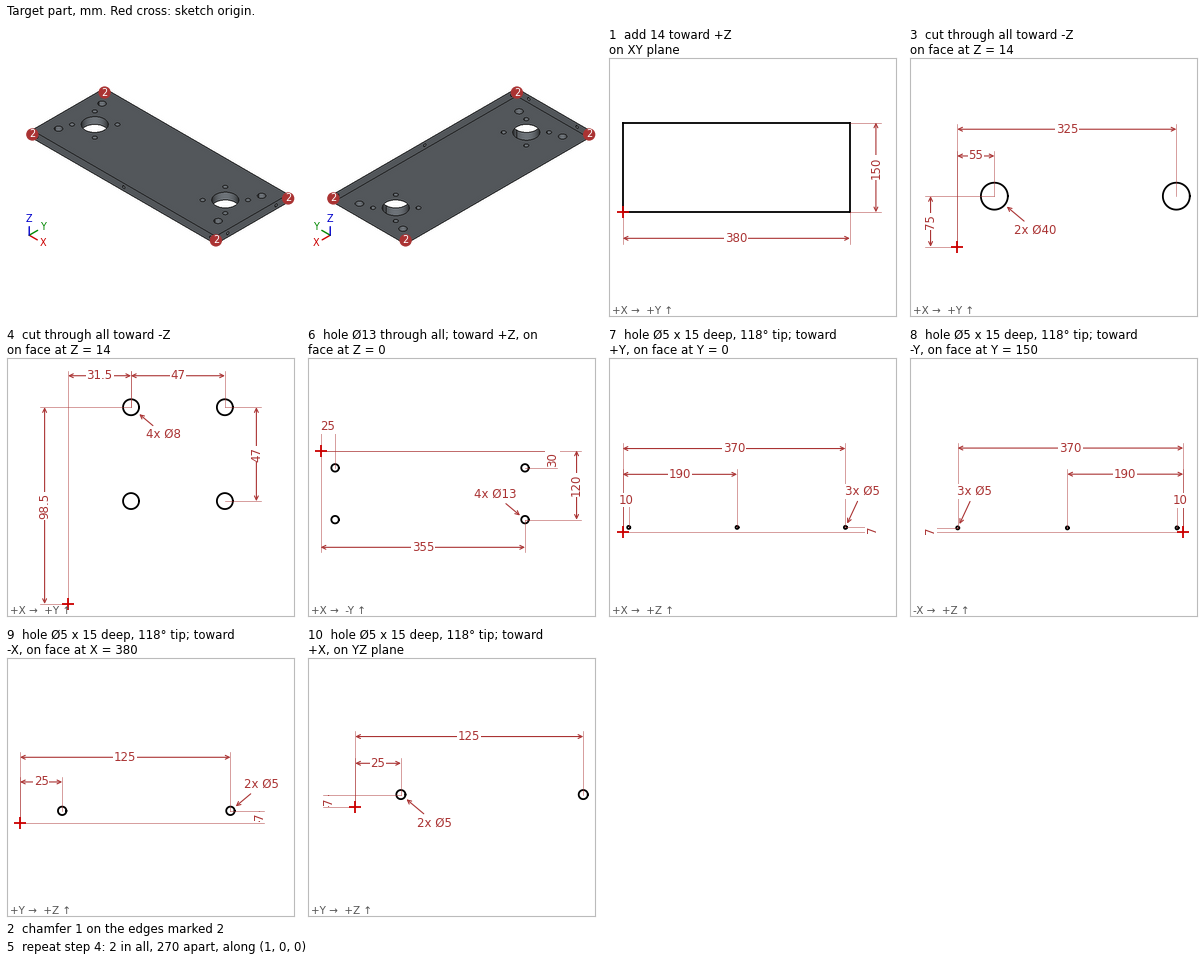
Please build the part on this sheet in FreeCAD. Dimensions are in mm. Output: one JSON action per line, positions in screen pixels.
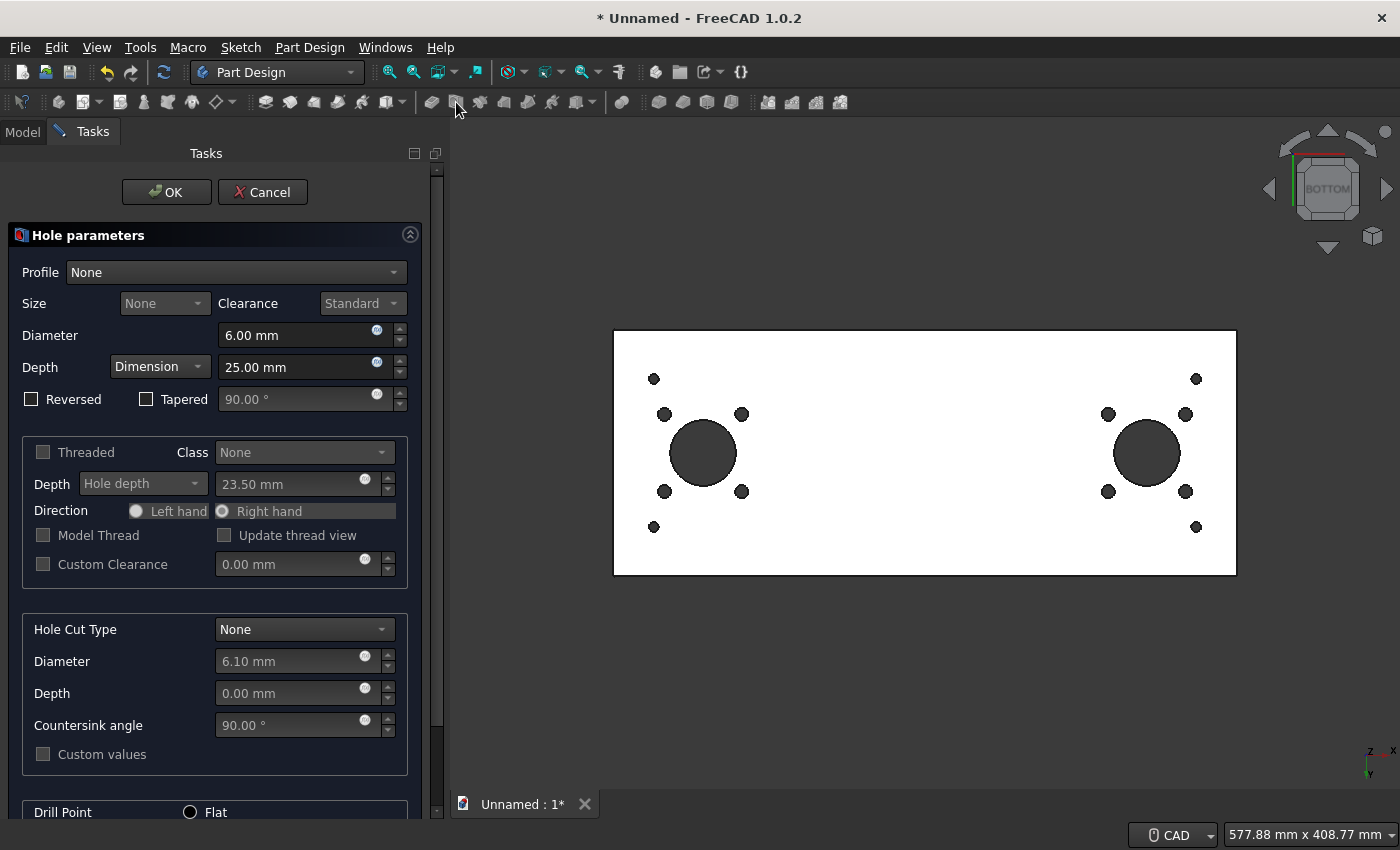
{"action": "triple_click", "coordinate": [305, 335]}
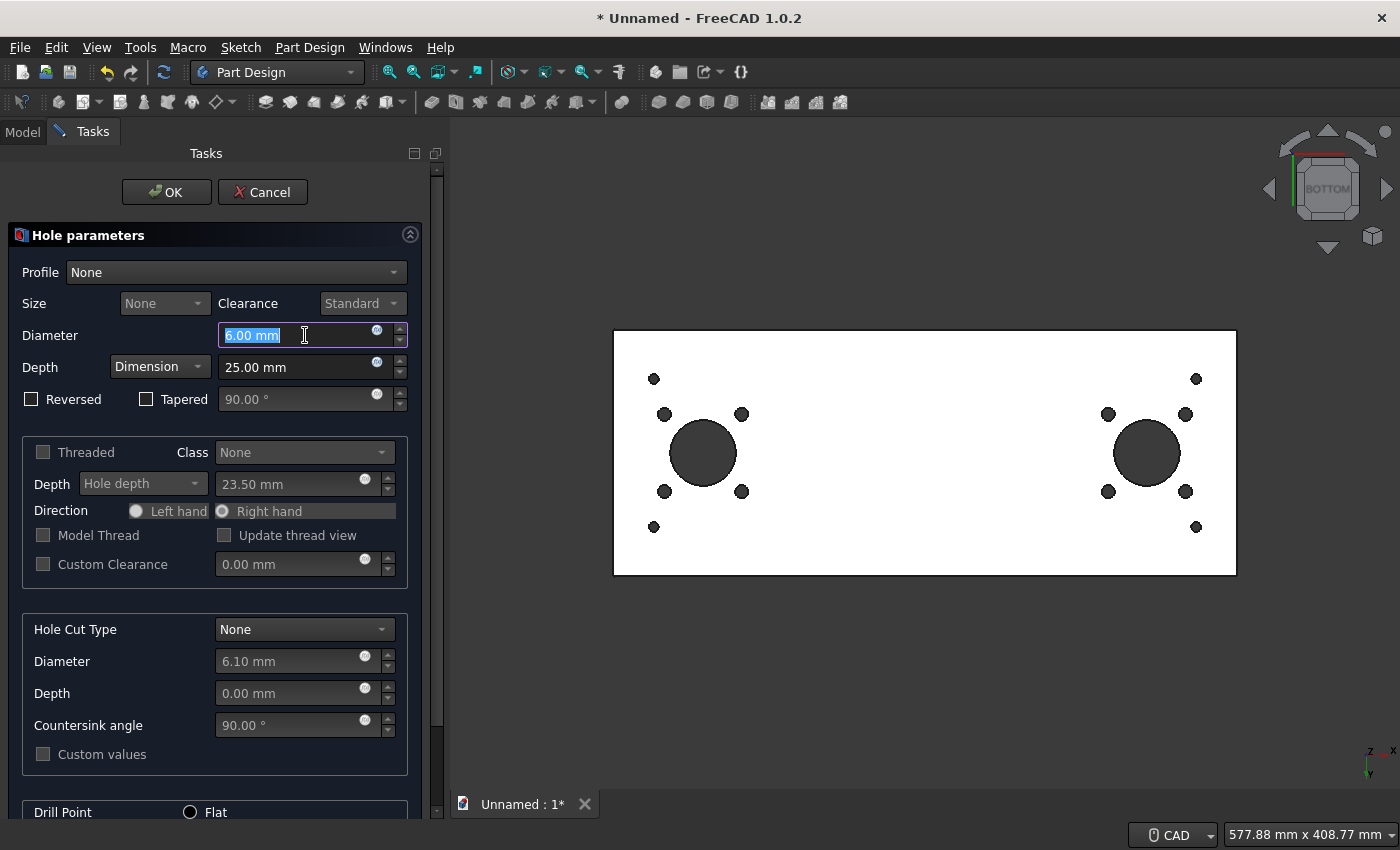
{"action": "type", "text": "13"}
{"action": "key", "text": "Tab"}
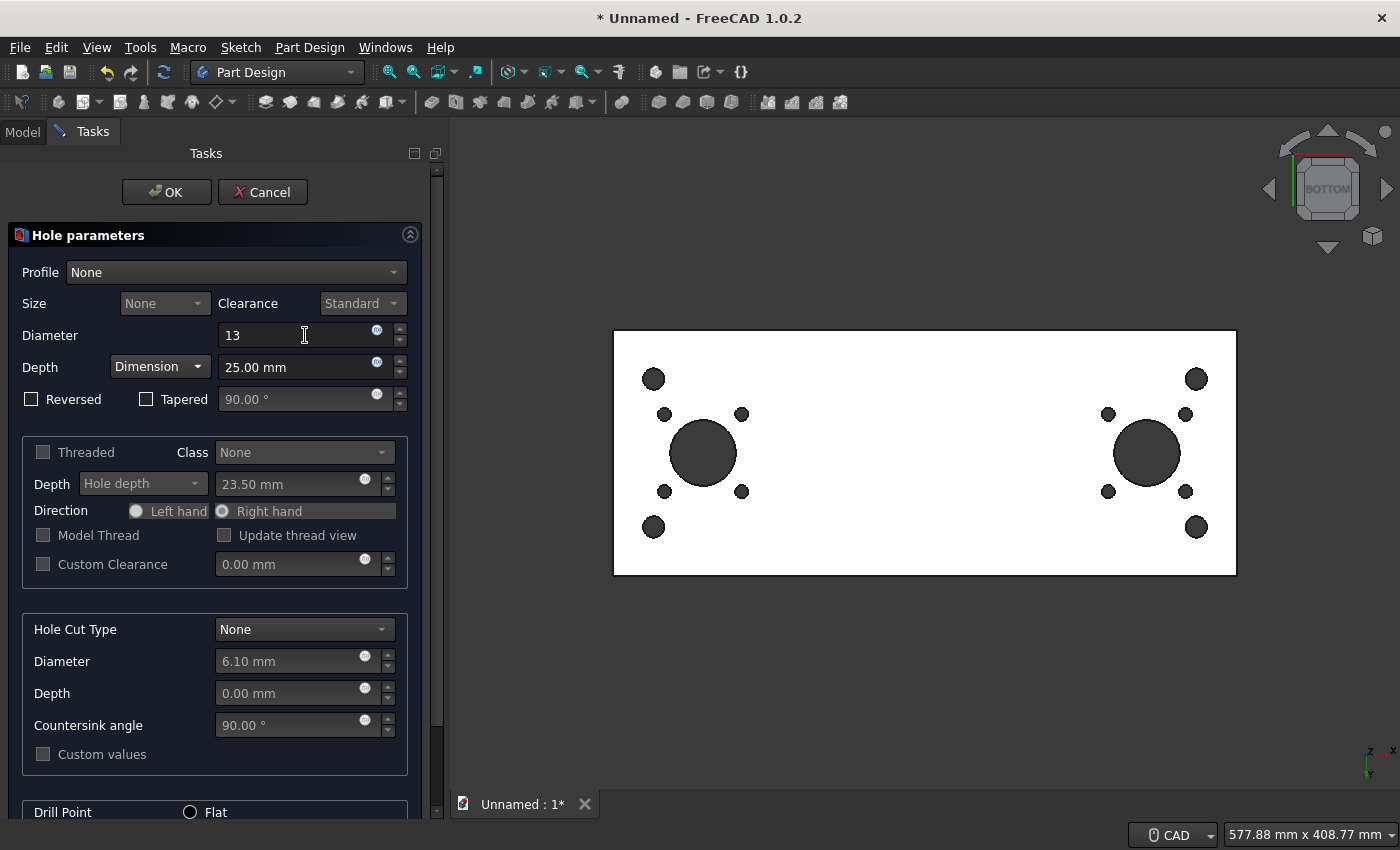
{"action": "left_click", "coordinate": [161, 366]}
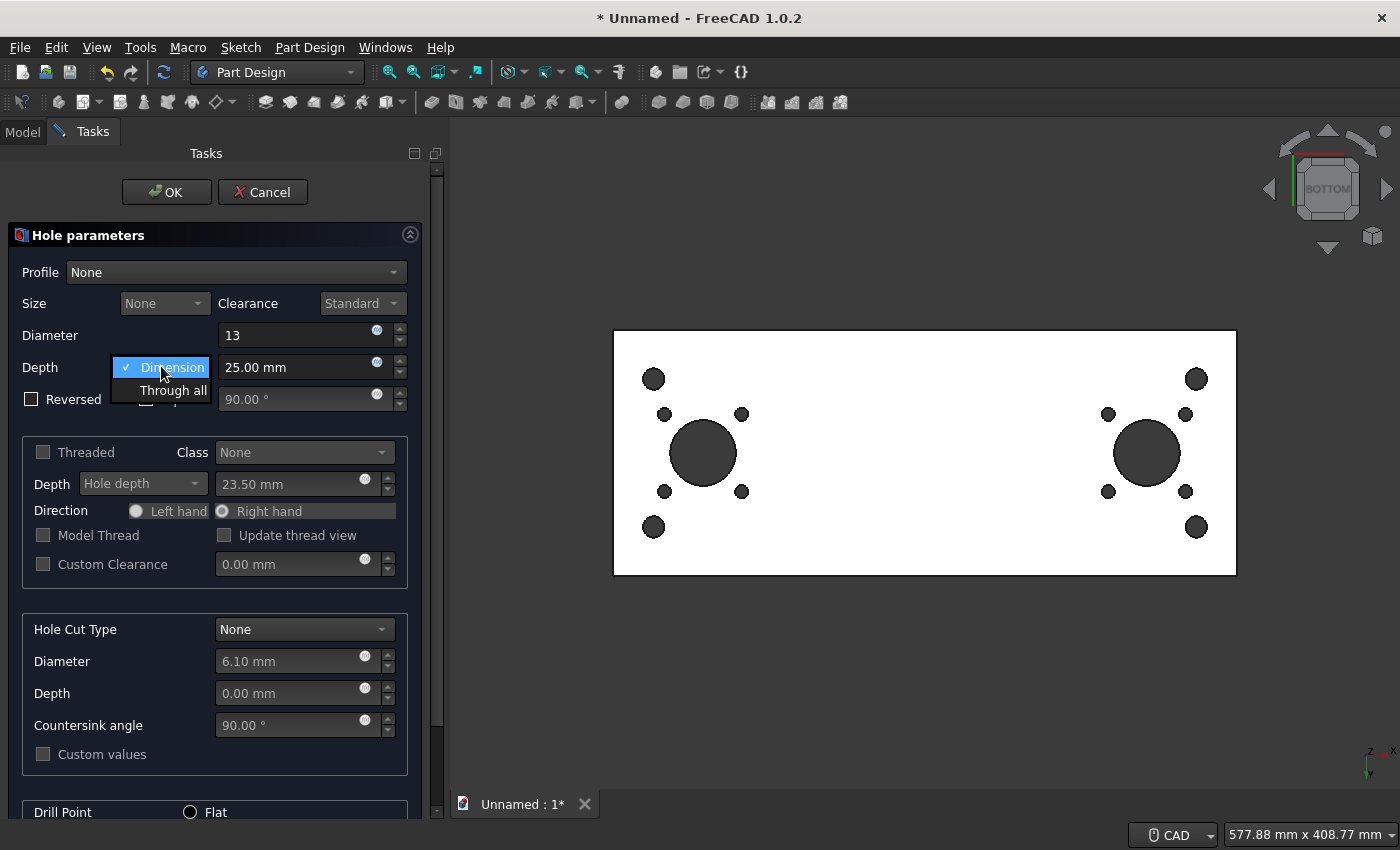
{"action": "left_click", "coordinate": [160, 390]}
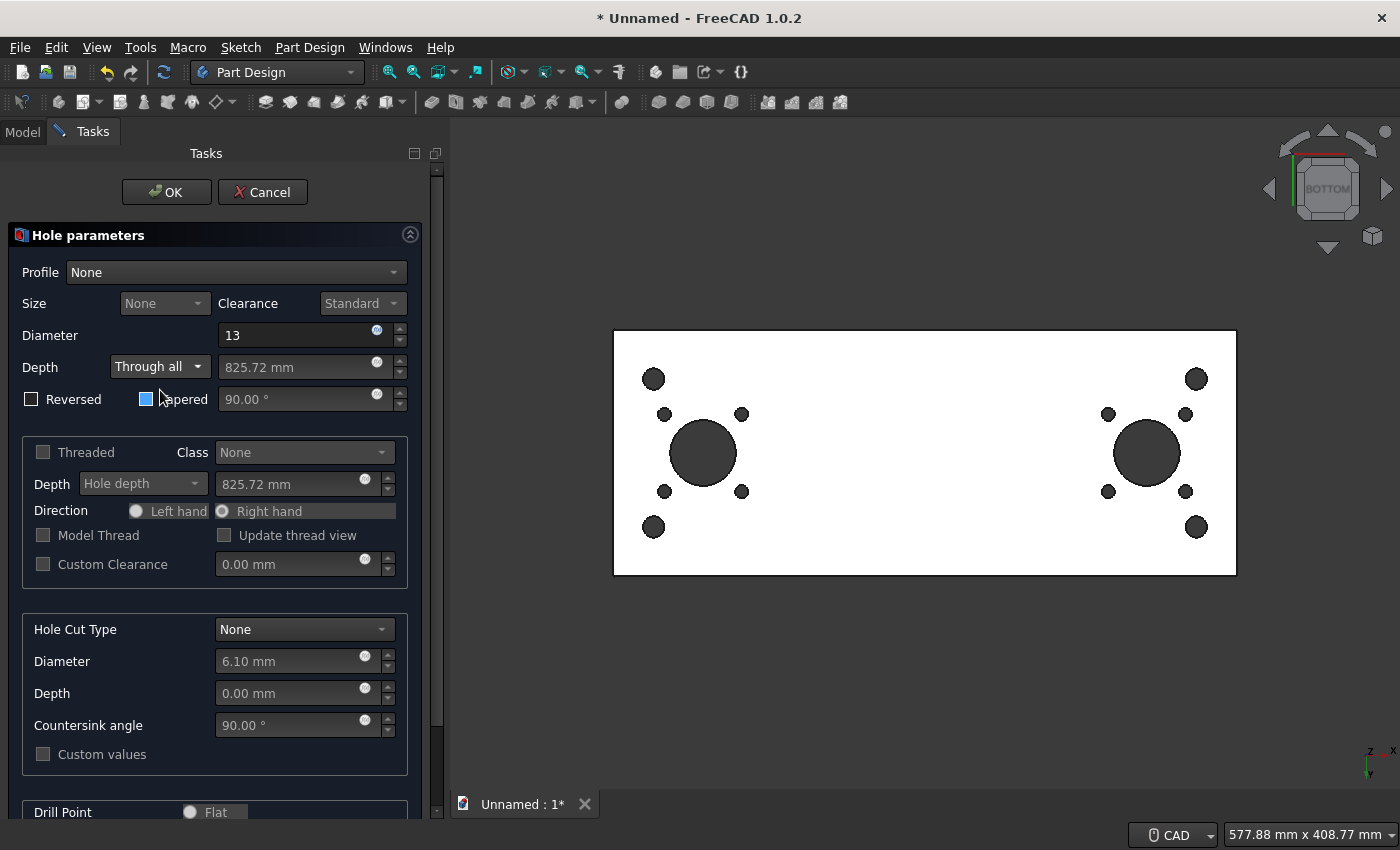
{"action": "left_click", "coordinate": [167, 192]}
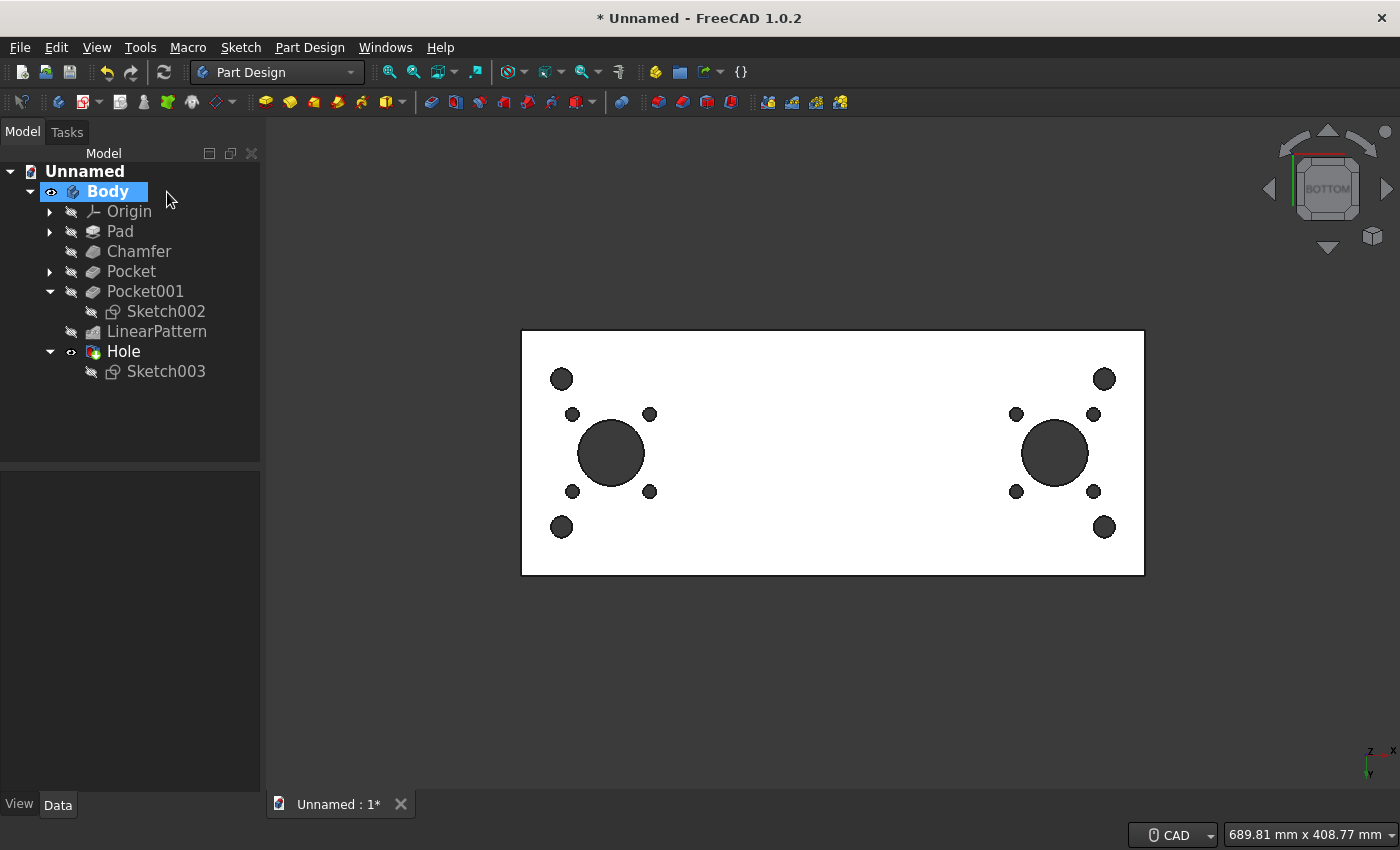
{"action": "key", "text": "0"}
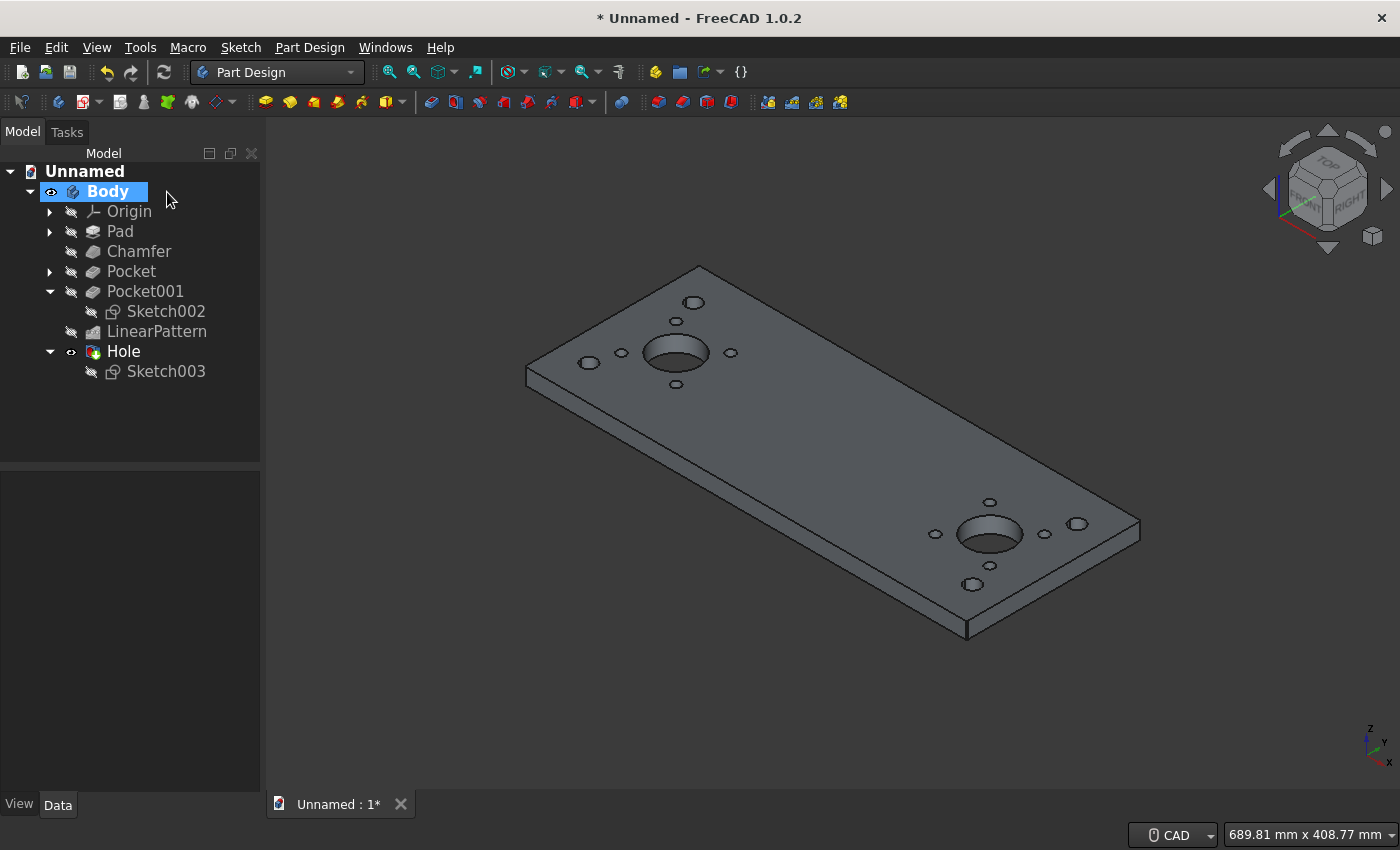
{"action": "key", "text": "1"}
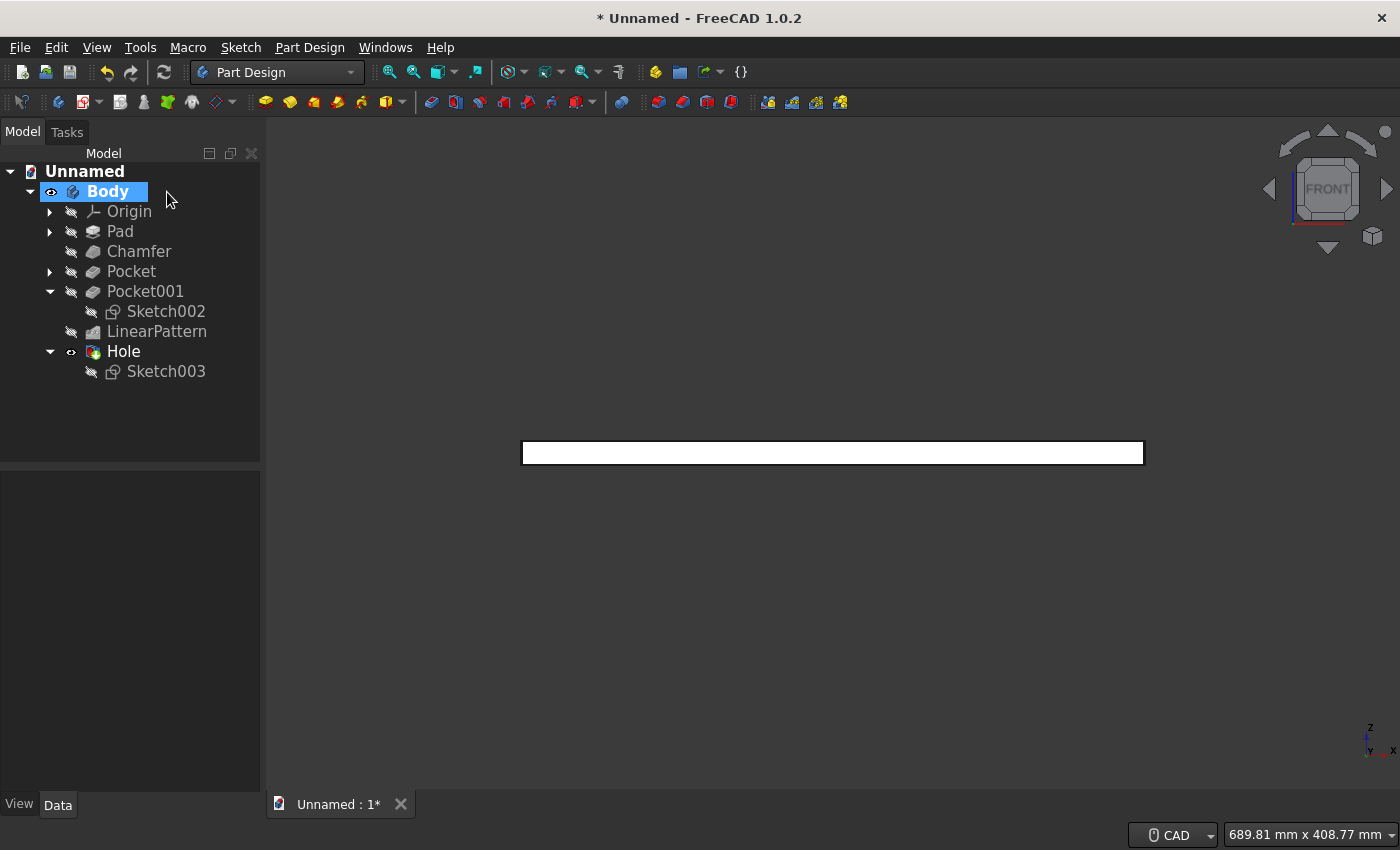
{"action": "left_click", "coordinate": [1099, 452]}